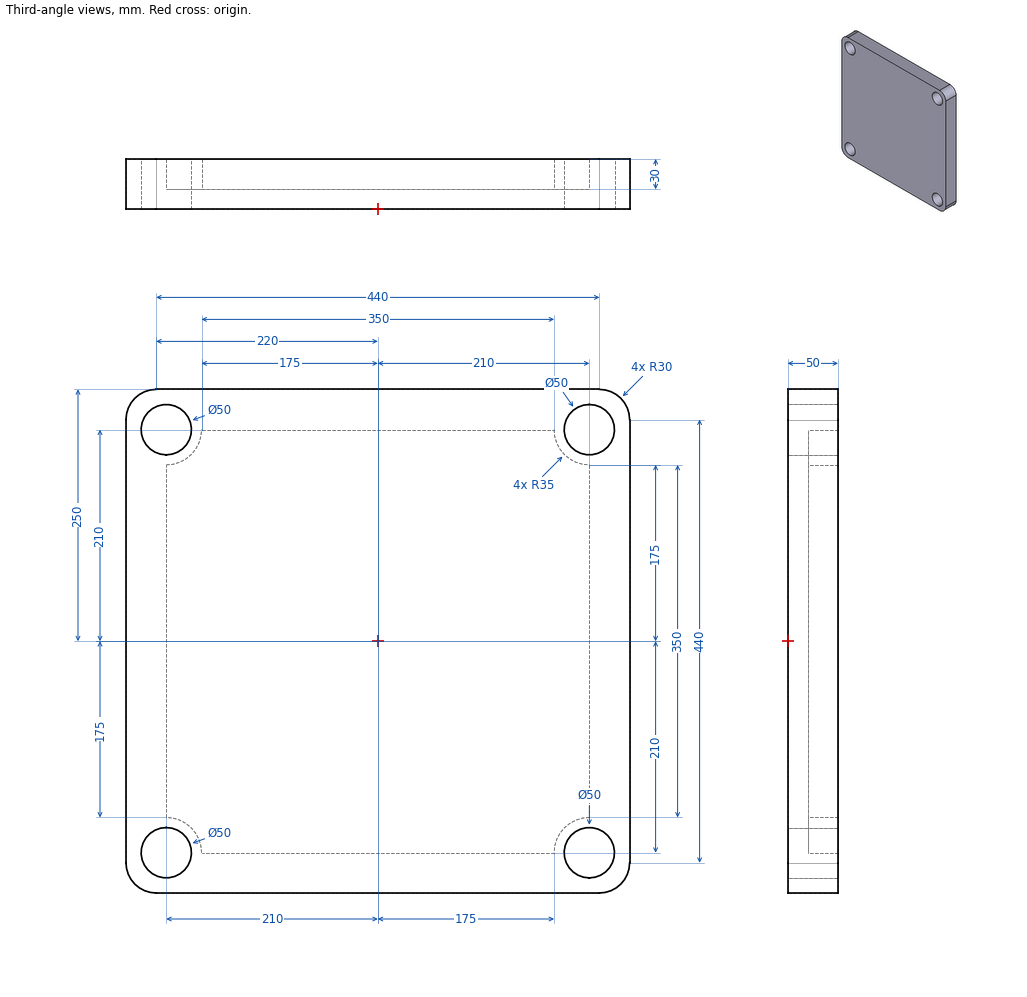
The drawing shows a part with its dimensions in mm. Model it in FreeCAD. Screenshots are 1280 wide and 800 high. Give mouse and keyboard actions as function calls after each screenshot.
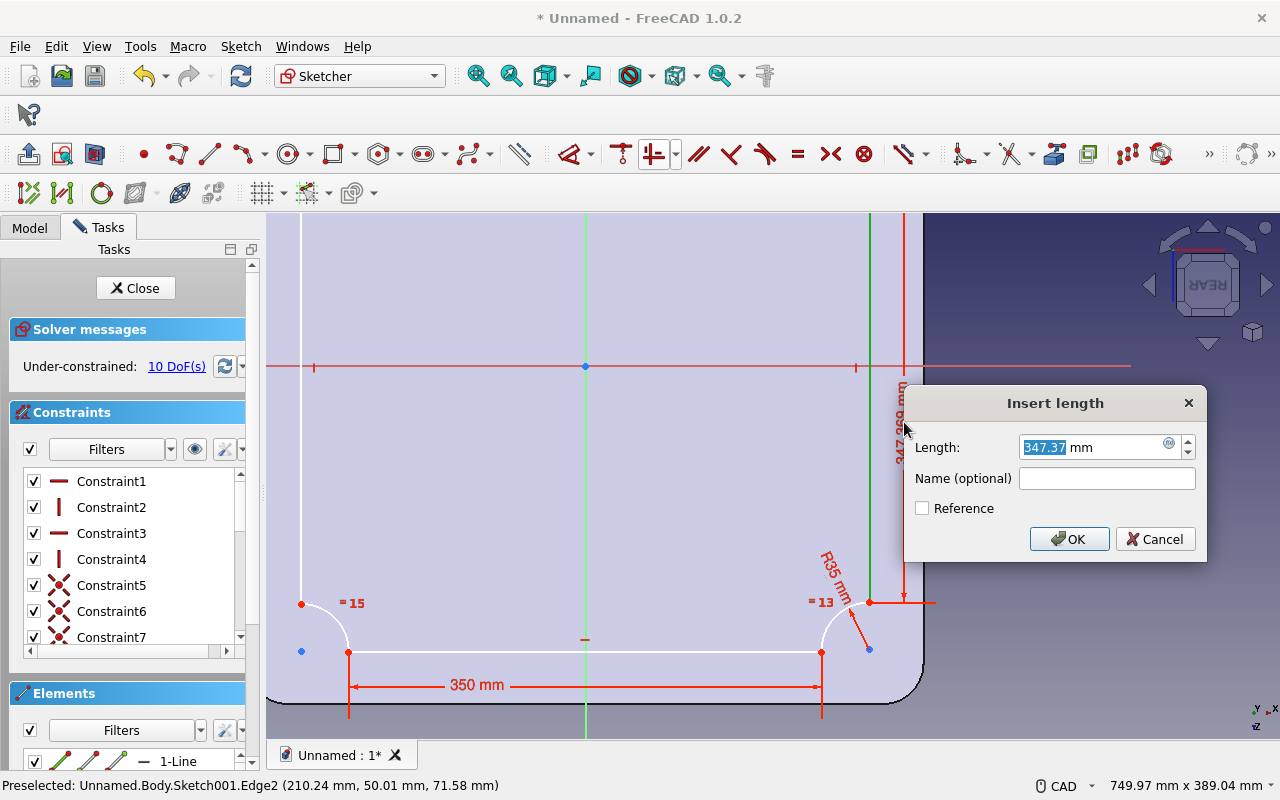
text(350)
key(Return)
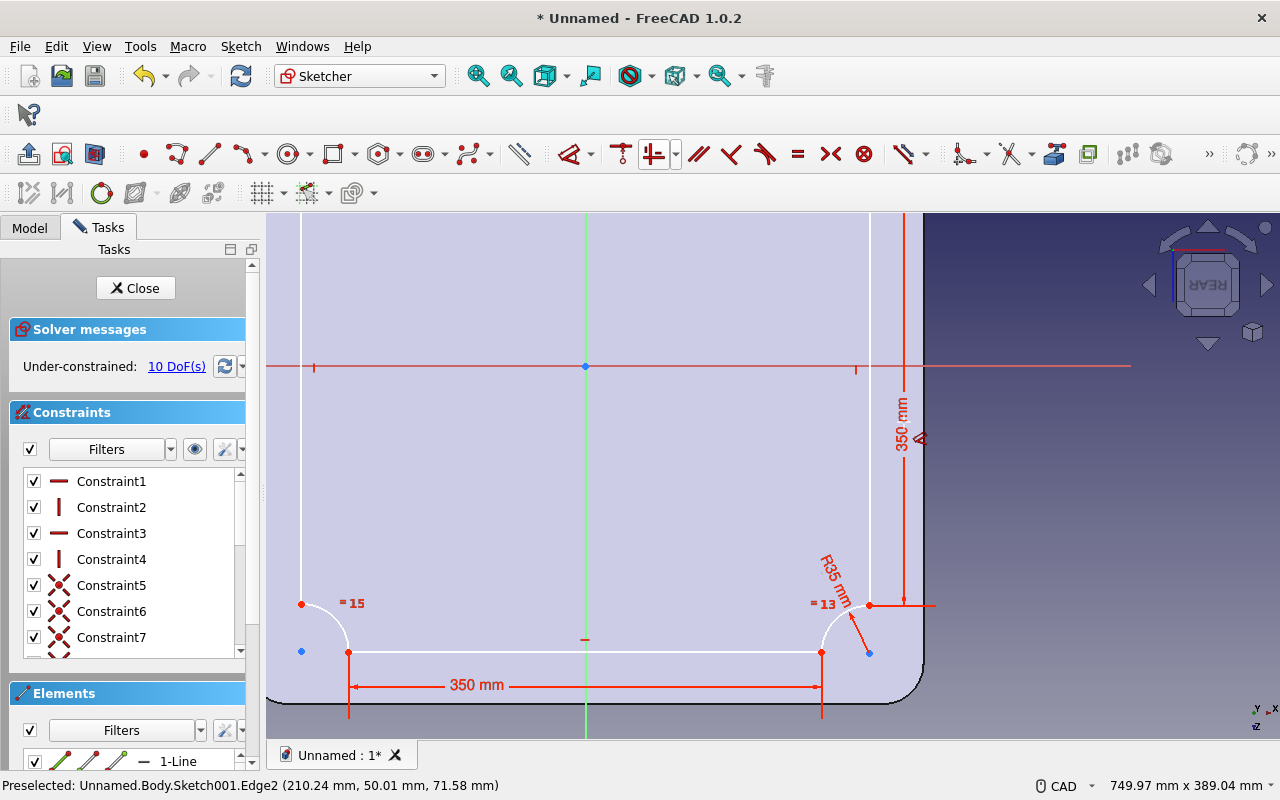
scroll(849, 610, down, 3)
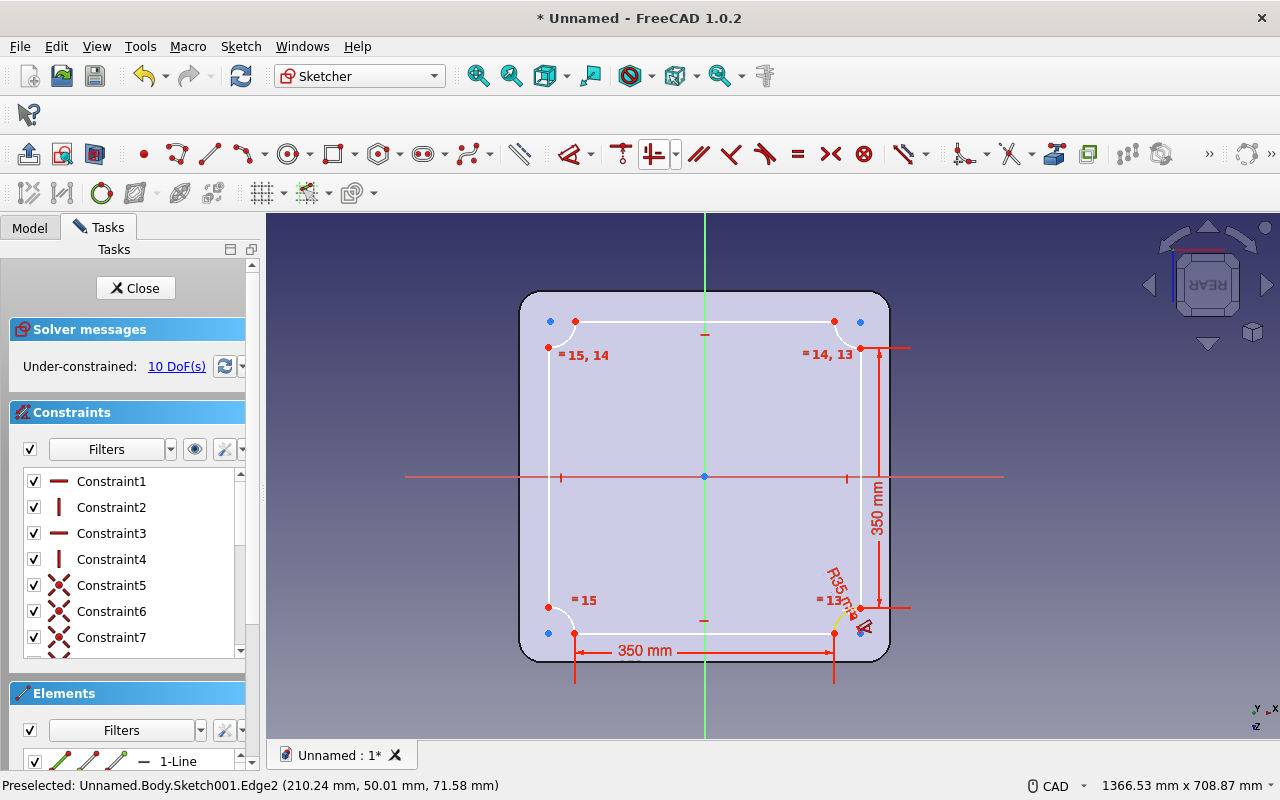
click(757, 322)
click(646, 288)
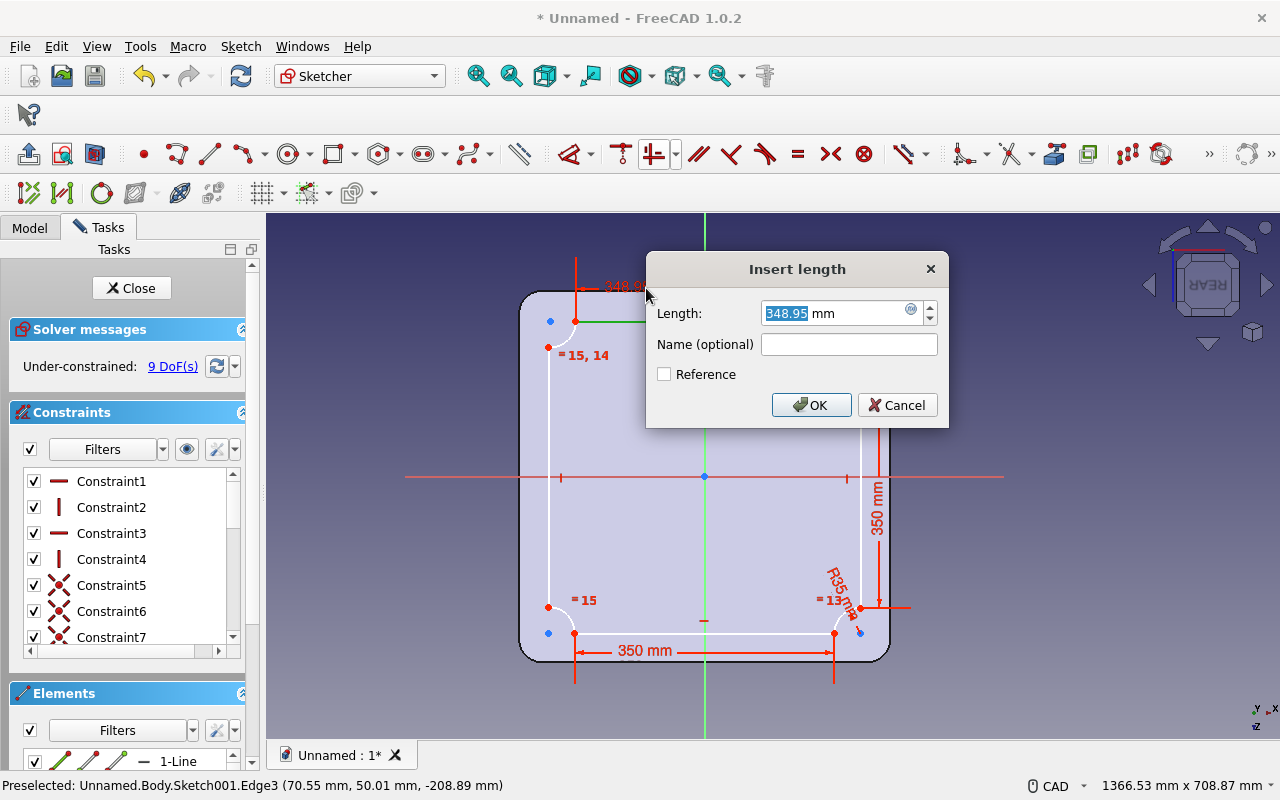
text(350)
key(Return)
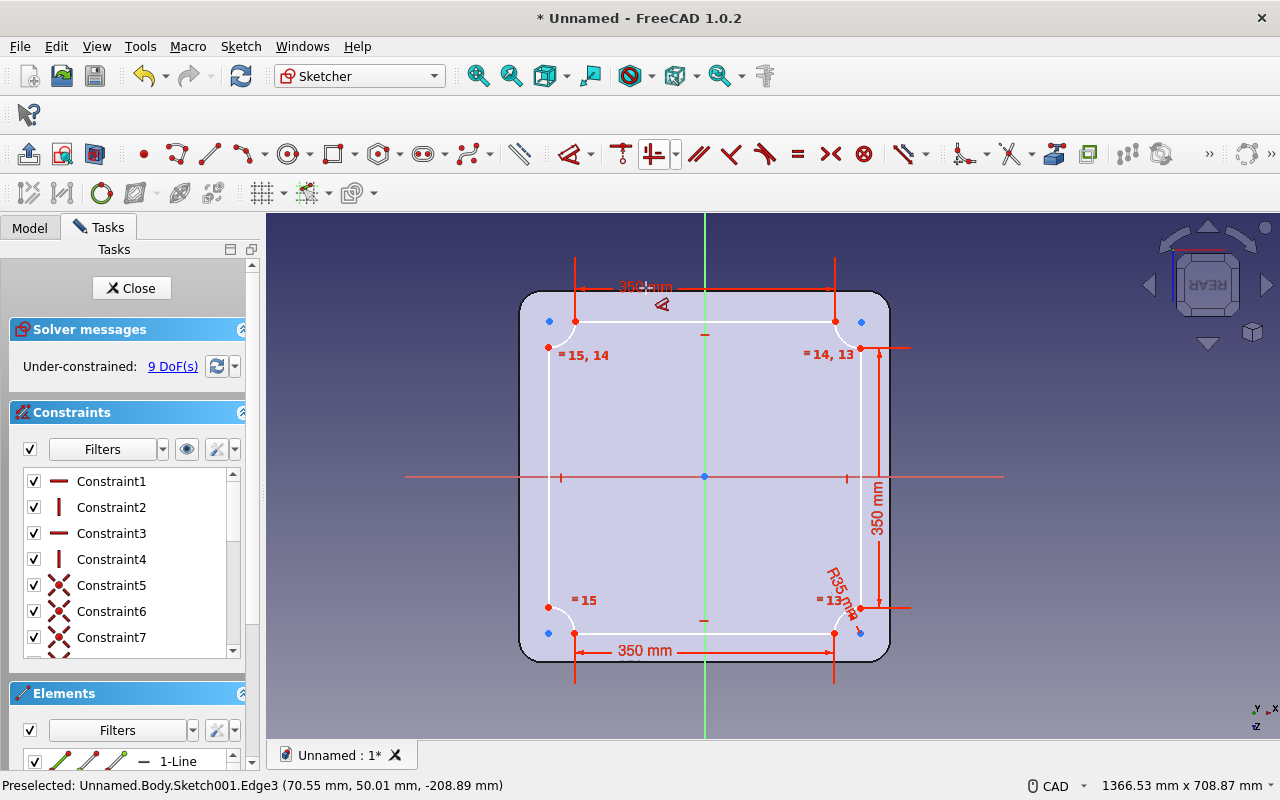
click(549, 425)
click(515, 417)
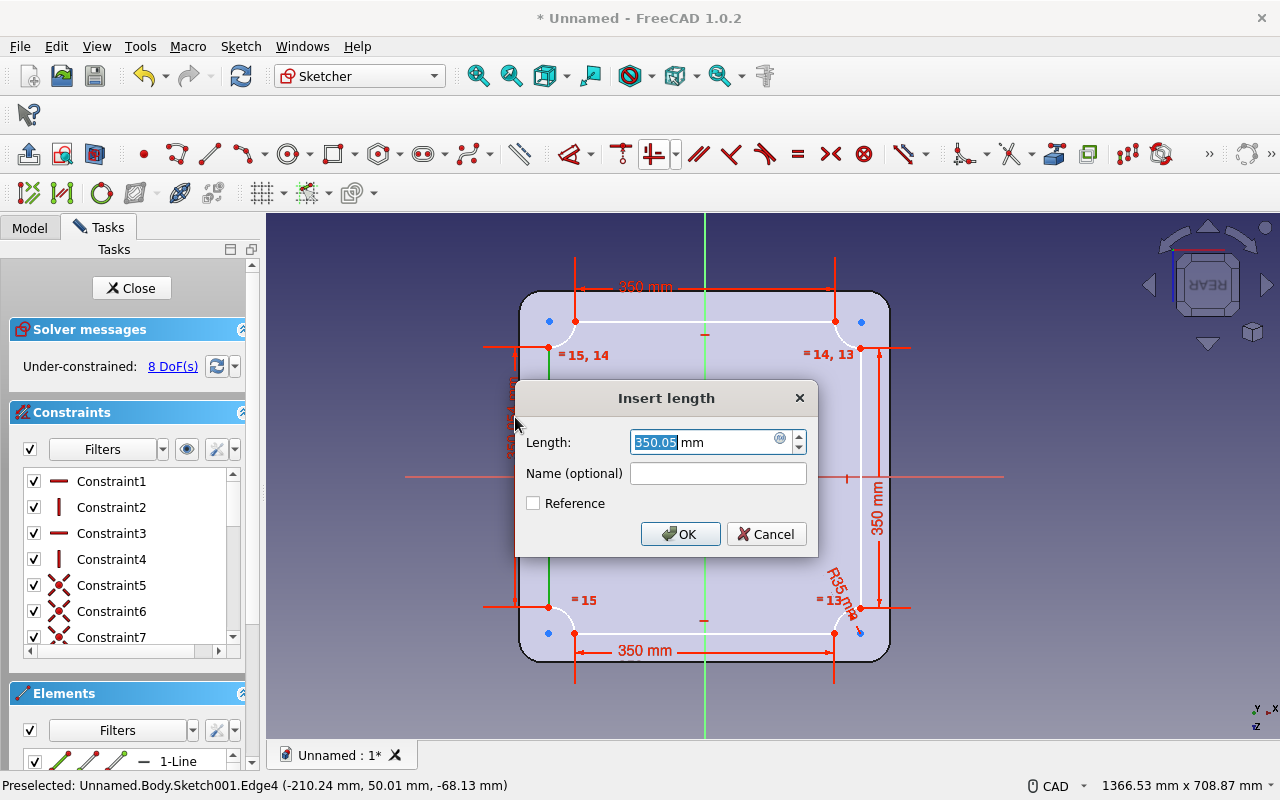
text(350)
key(Return)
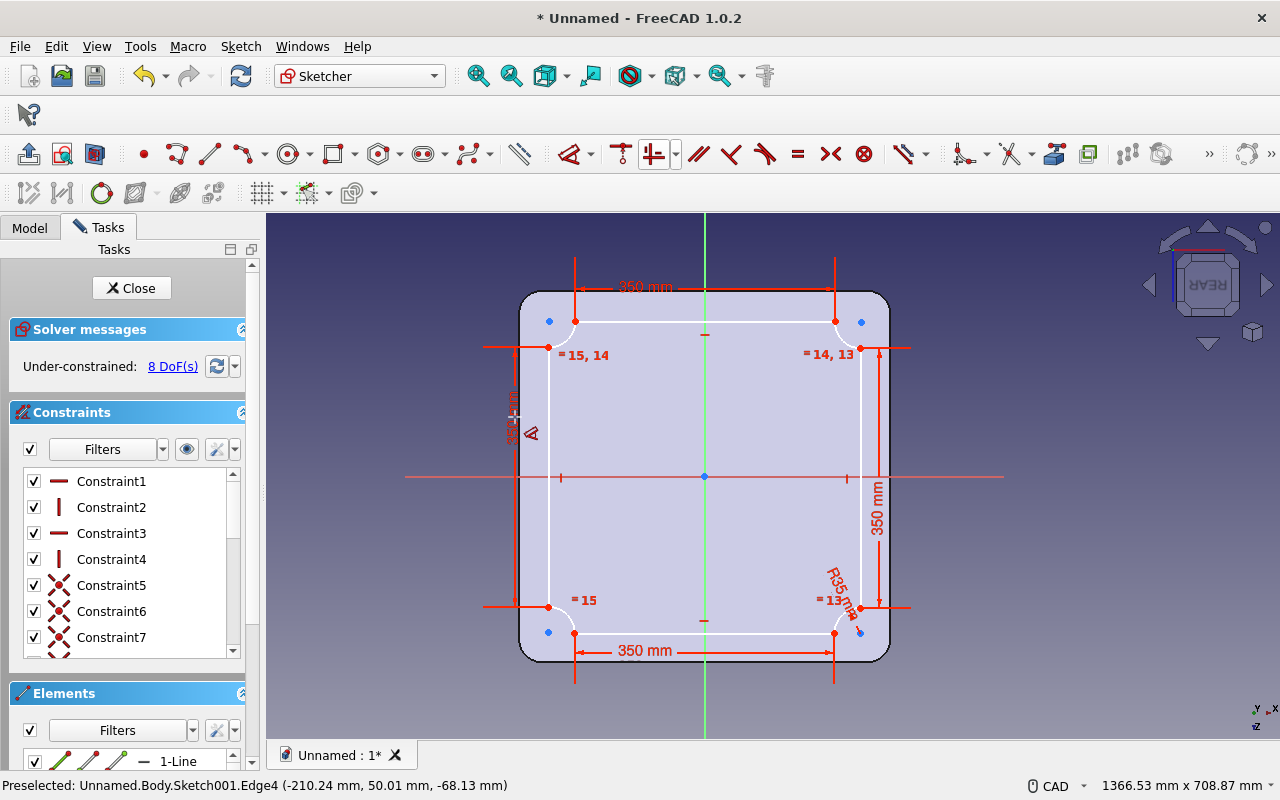
click(575, 634)
click(640, 443)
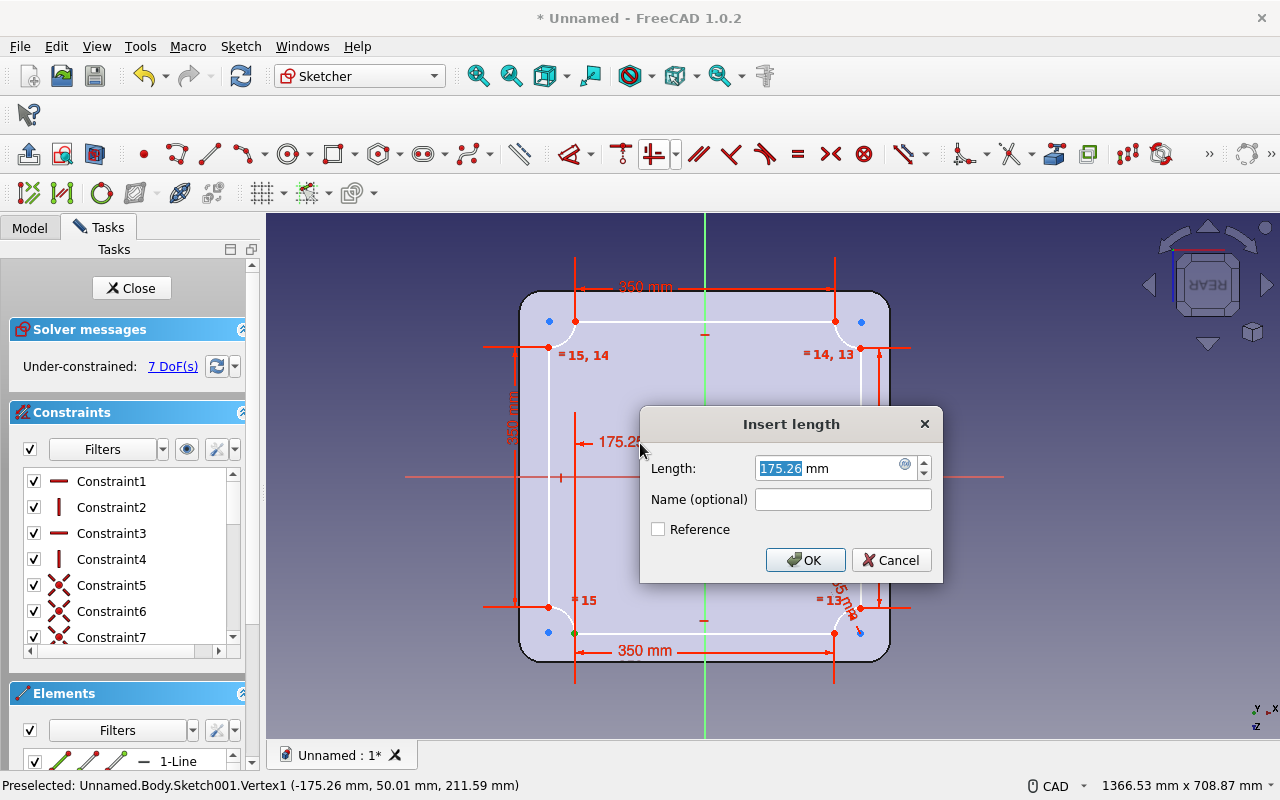
text(175)
key(Return)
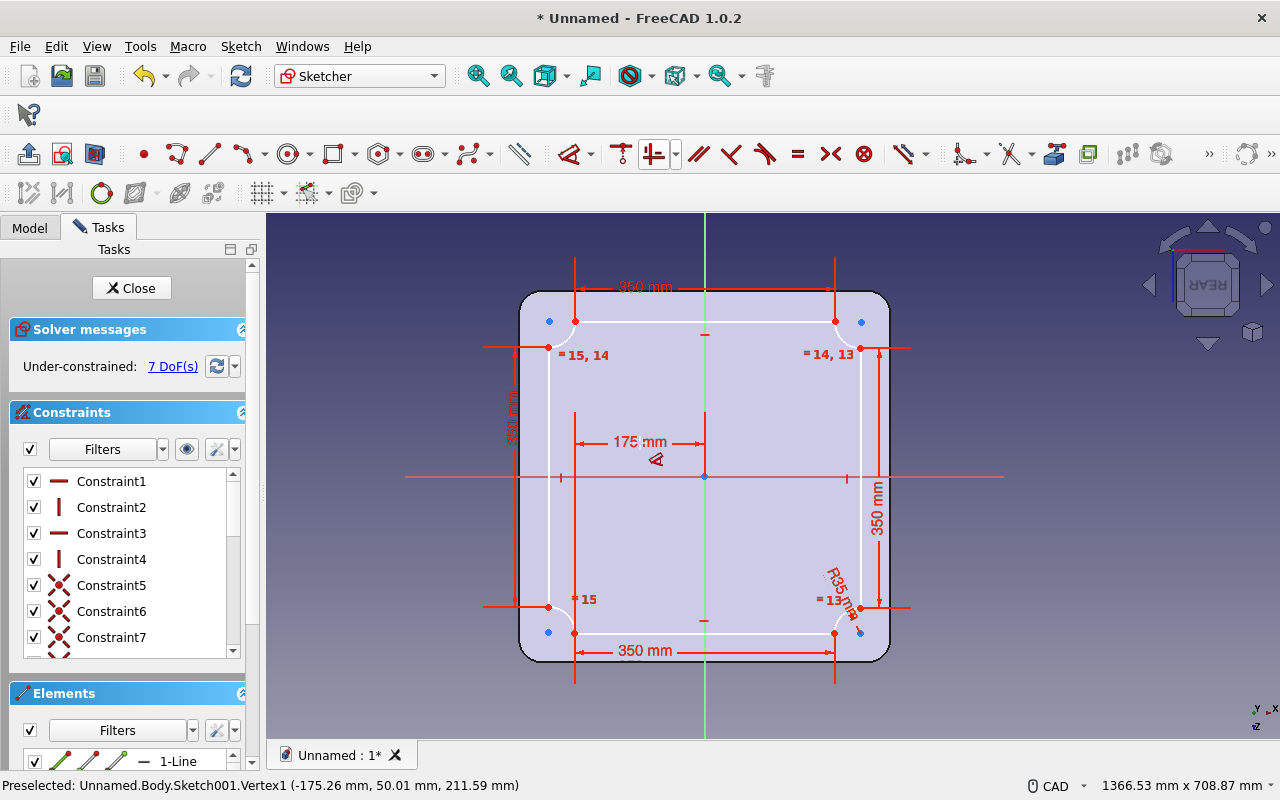
click(575, 634)
click(739, 555)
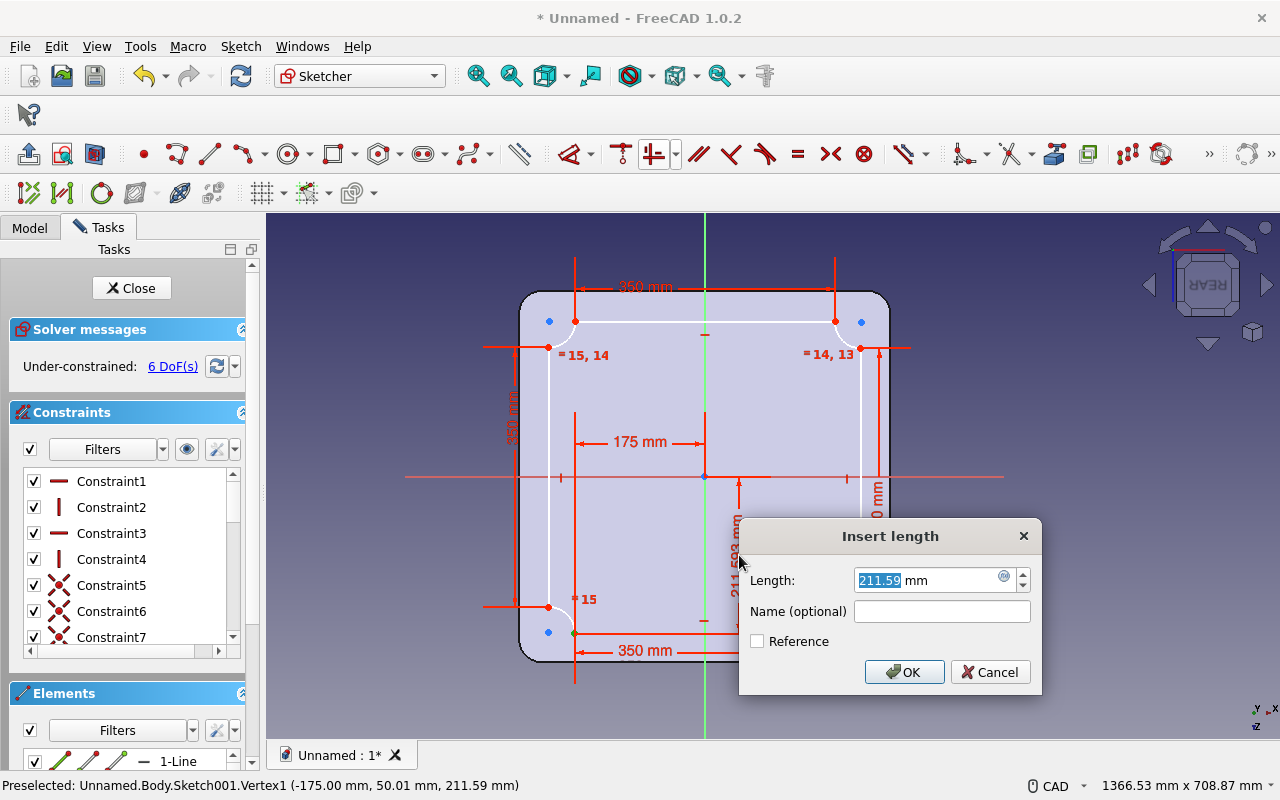
text(210)
key(Return)